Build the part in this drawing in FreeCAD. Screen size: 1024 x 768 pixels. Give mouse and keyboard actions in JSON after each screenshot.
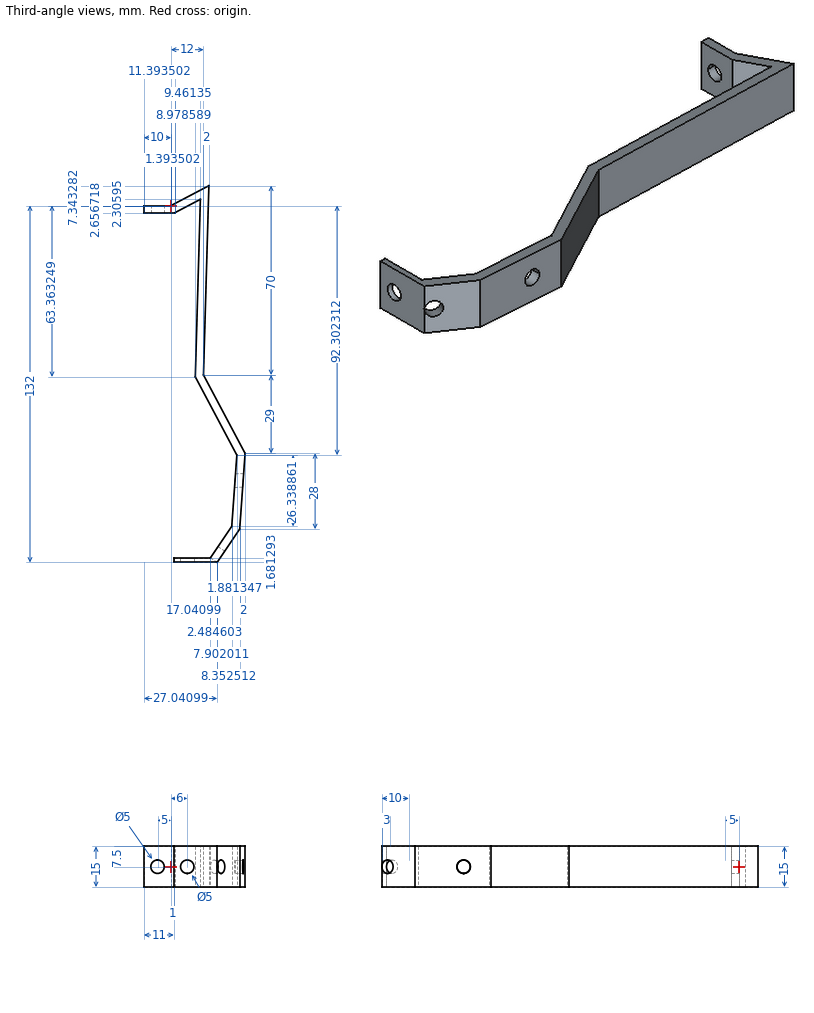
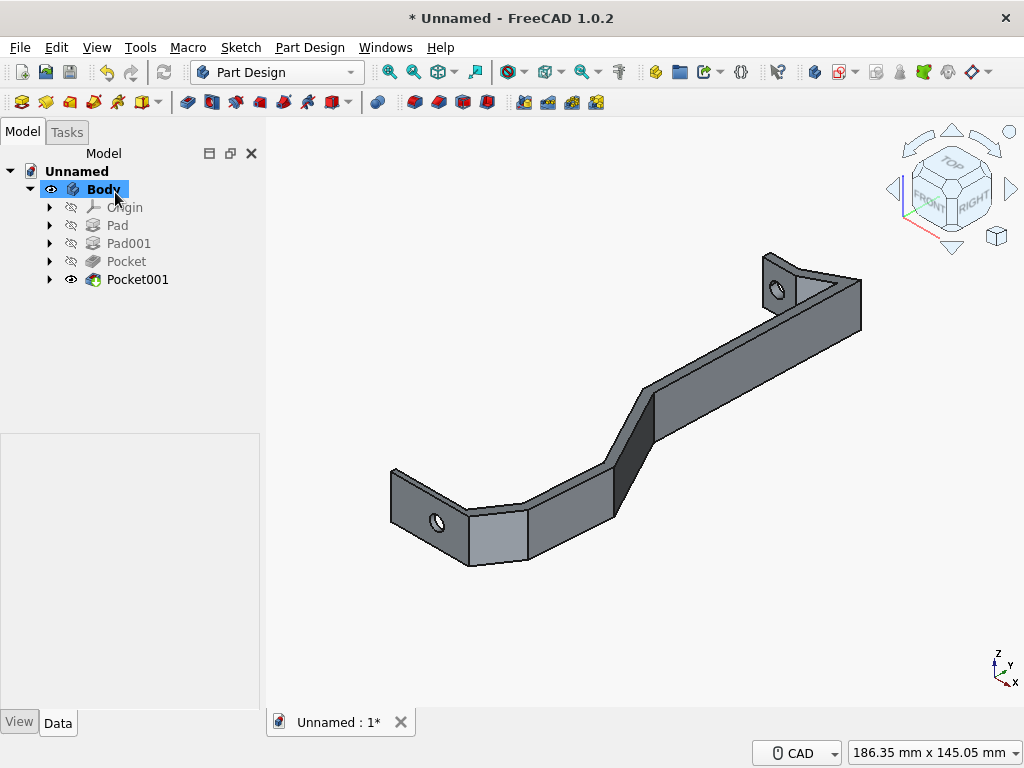
{"action": "left_click", "coordinate": [408, 505]}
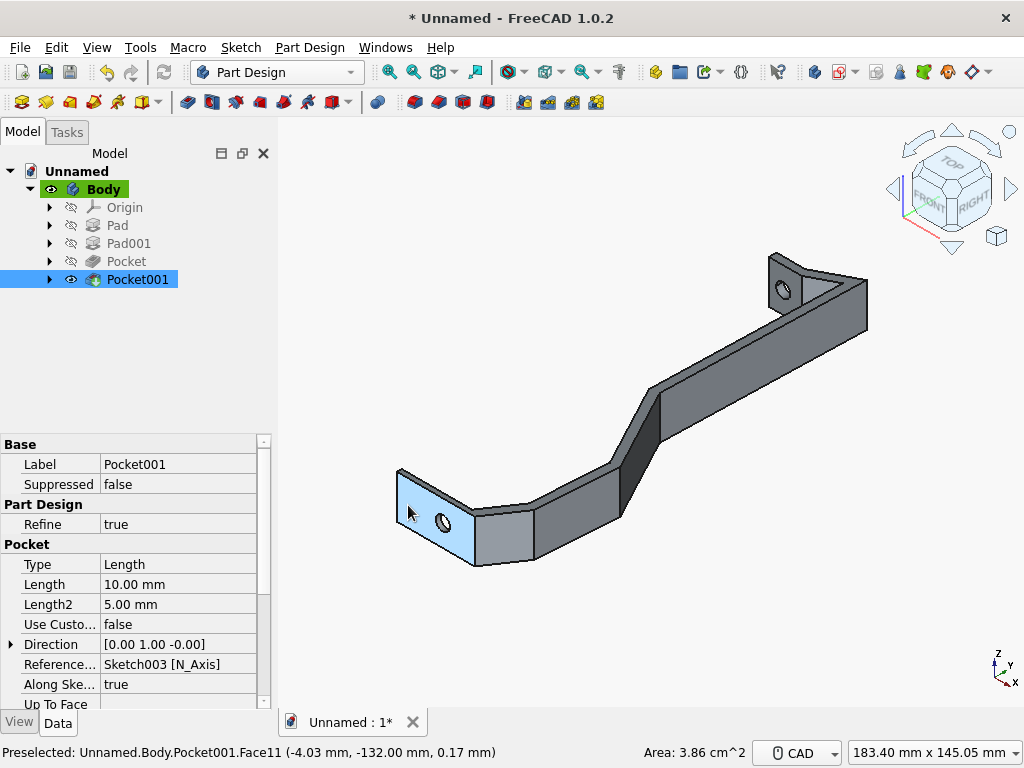
{"action": "left_click", "coordinate": [840, 72]}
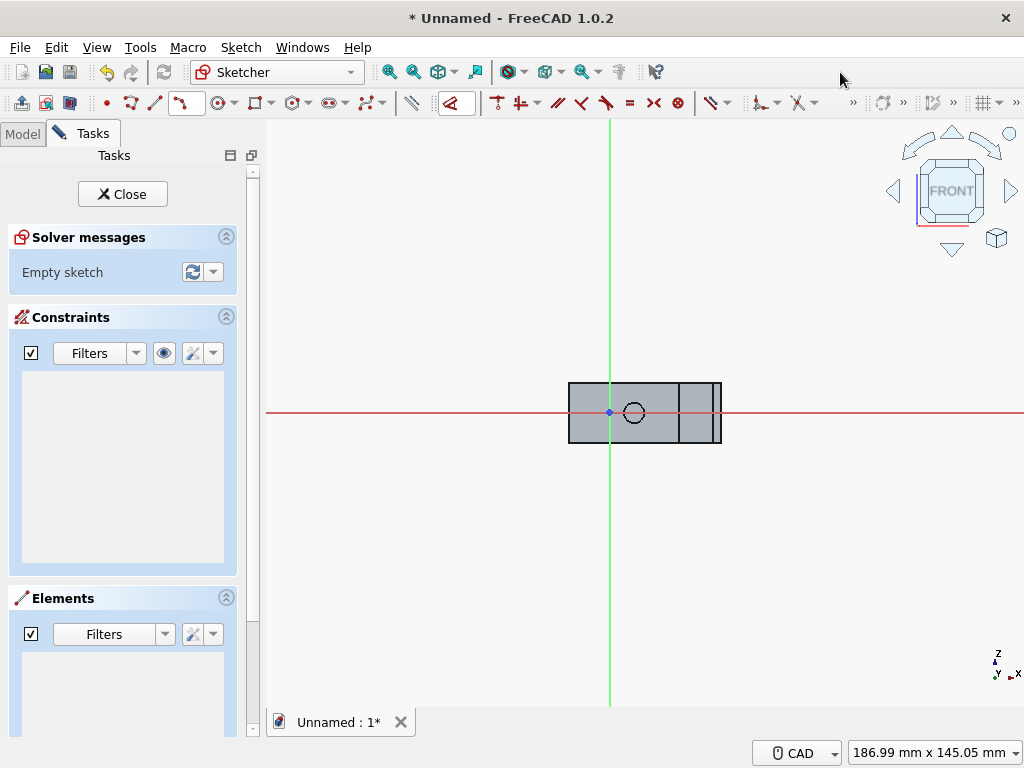
{"action": "scroll", "coordinate": [594, 413], "scroll_direction": "up", "scroll_amount": 9}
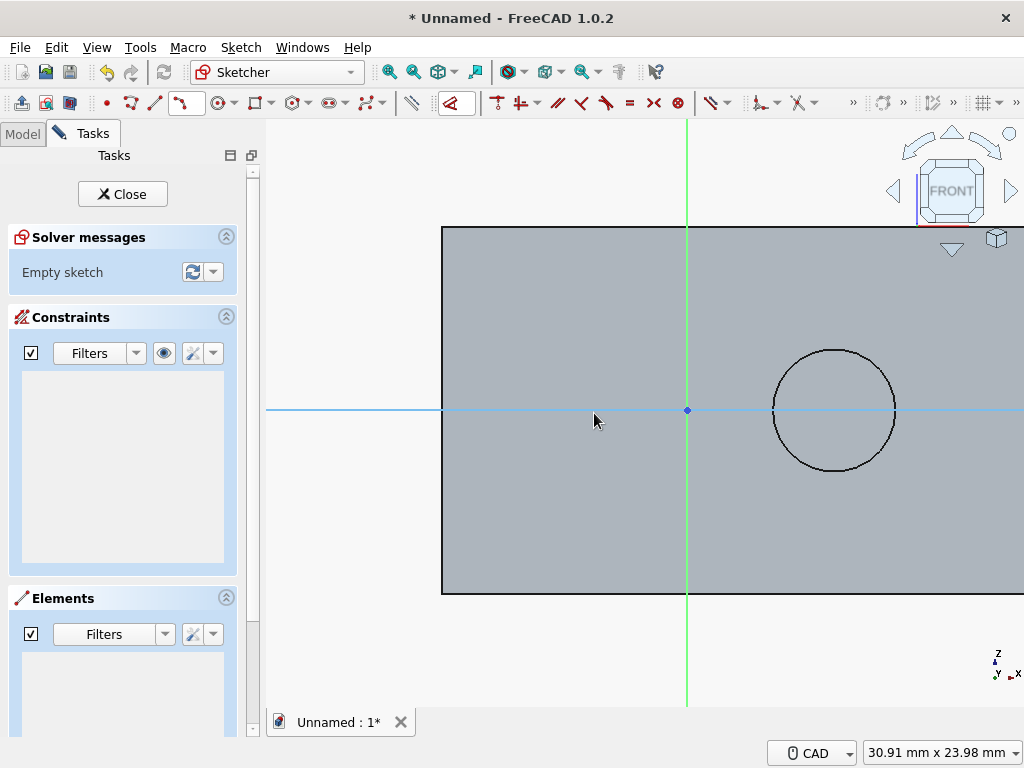
{"action": "left_click", "coordinate": [256, 104]}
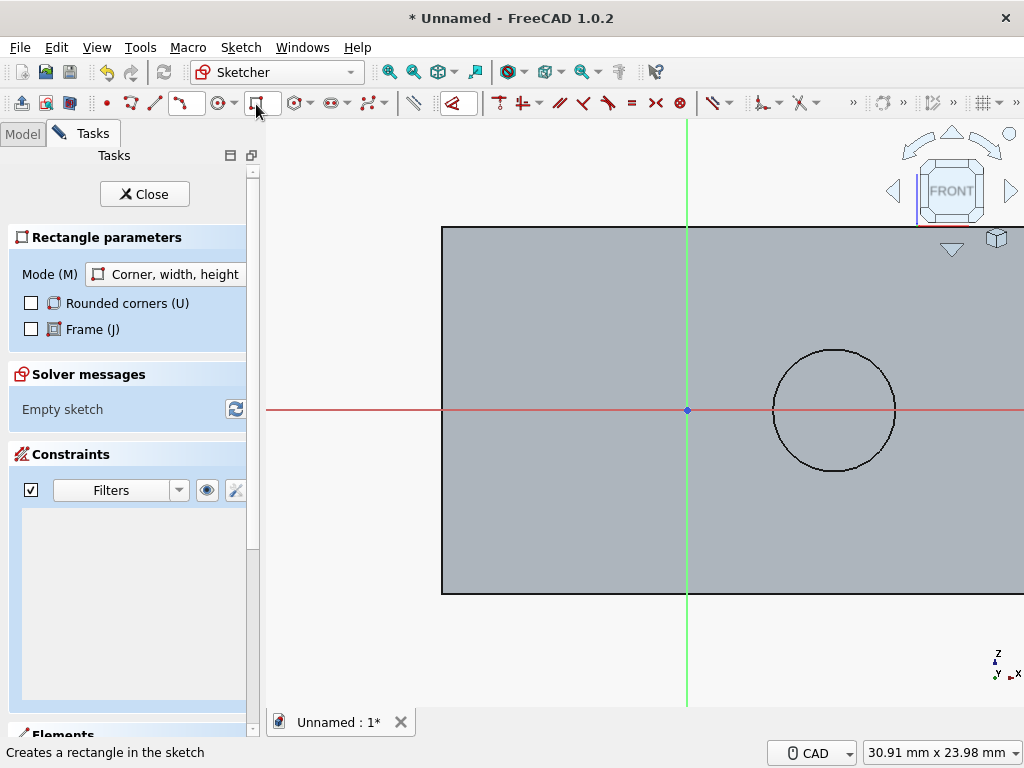
{"action": "left_click", "coordinate": [442, 227]}
{"action": "mouse_move", "coordinate": [712, 594]}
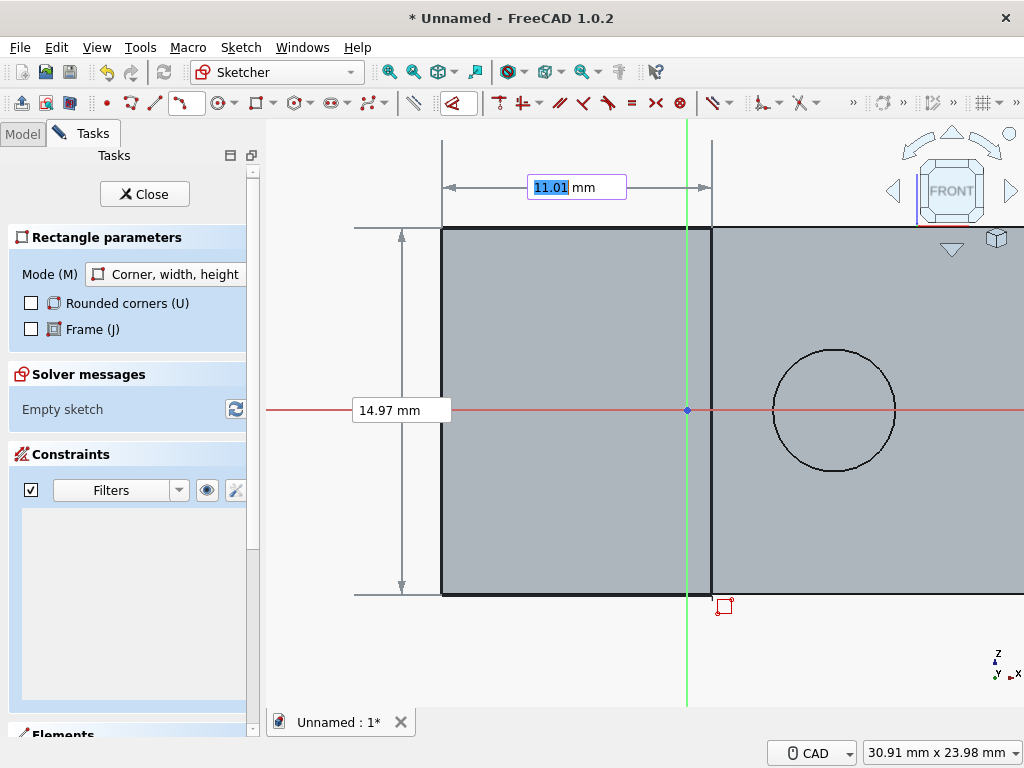
{"action": "type", "text": "11"}
{"action": "key", "text": "Tab"}
{"action": "type", "text": "15"}
{"action": "key", "text": "Return"}
{"action": "key", "text": "Escape"}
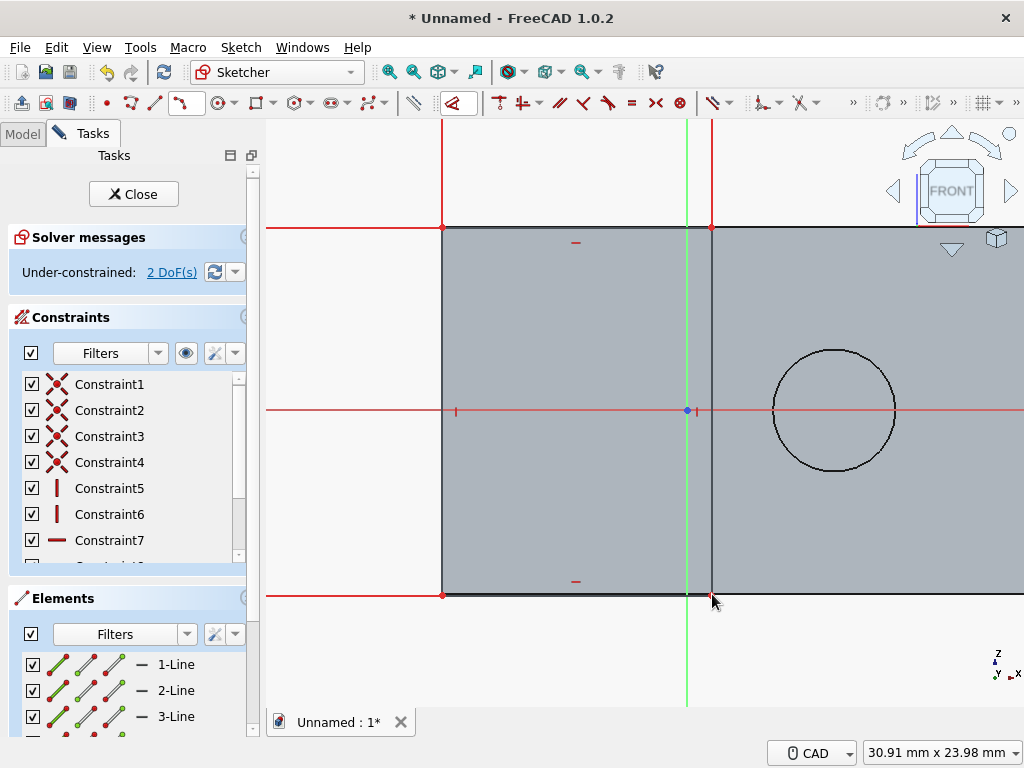
{"action": "scroll", "coordinate": [712, 596], "scroll_direction": "up", "scroll_amount": 3}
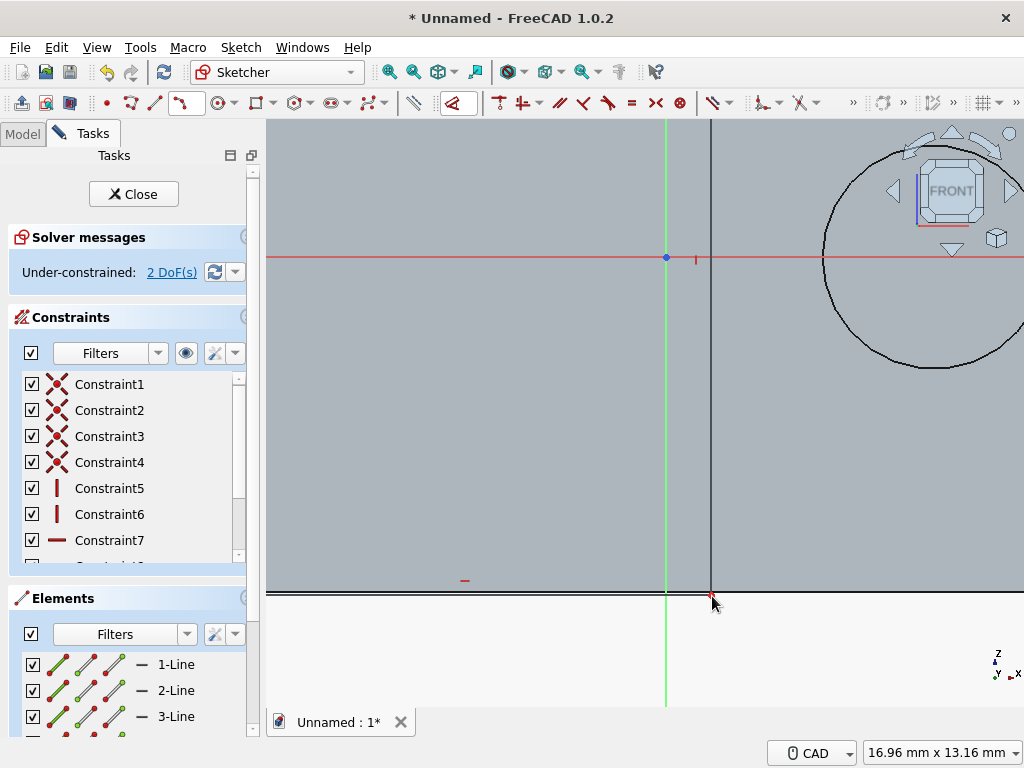
{"action": "left_click", "coordinate": [711, 595]}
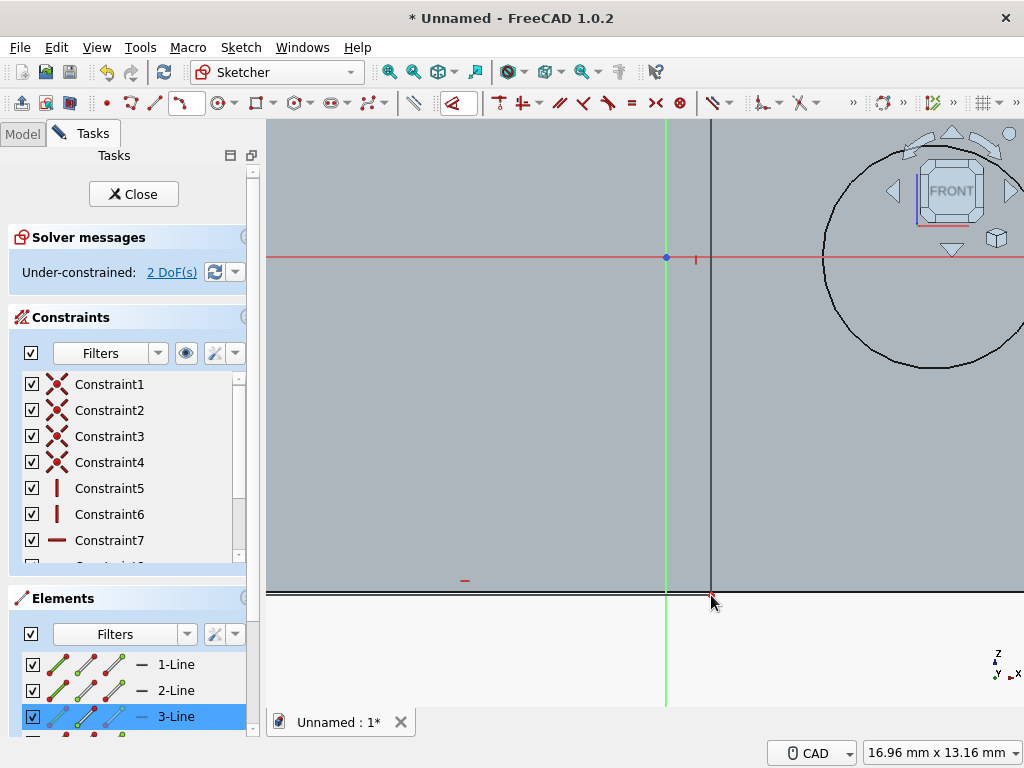
{"action": "left_click", "coordinate": [472, 104]}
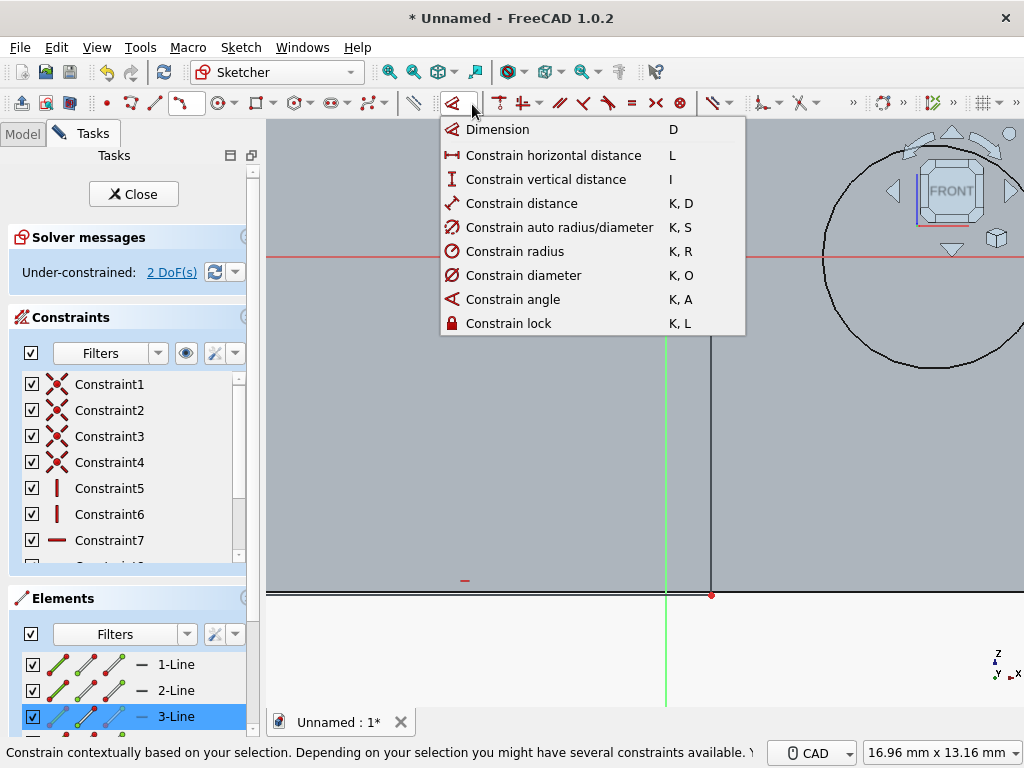
{"action": "left_click", "coordinate": [593, 155]}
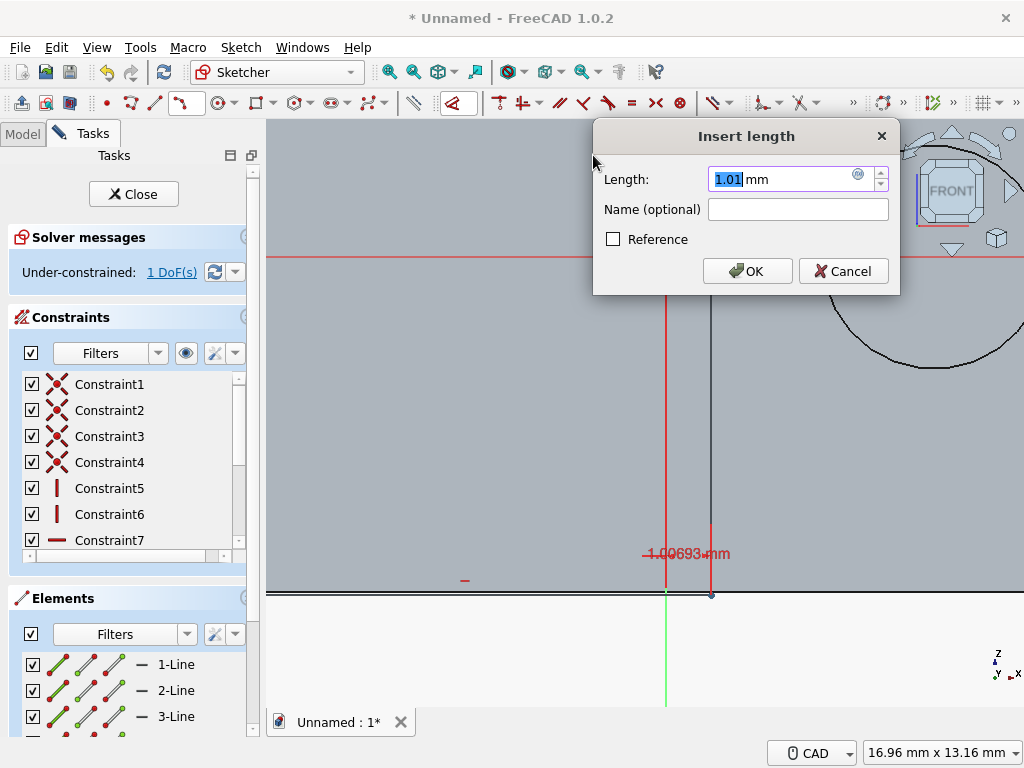
{"action": "type", "text": "1"}
{"action": "key", "text": "Return"}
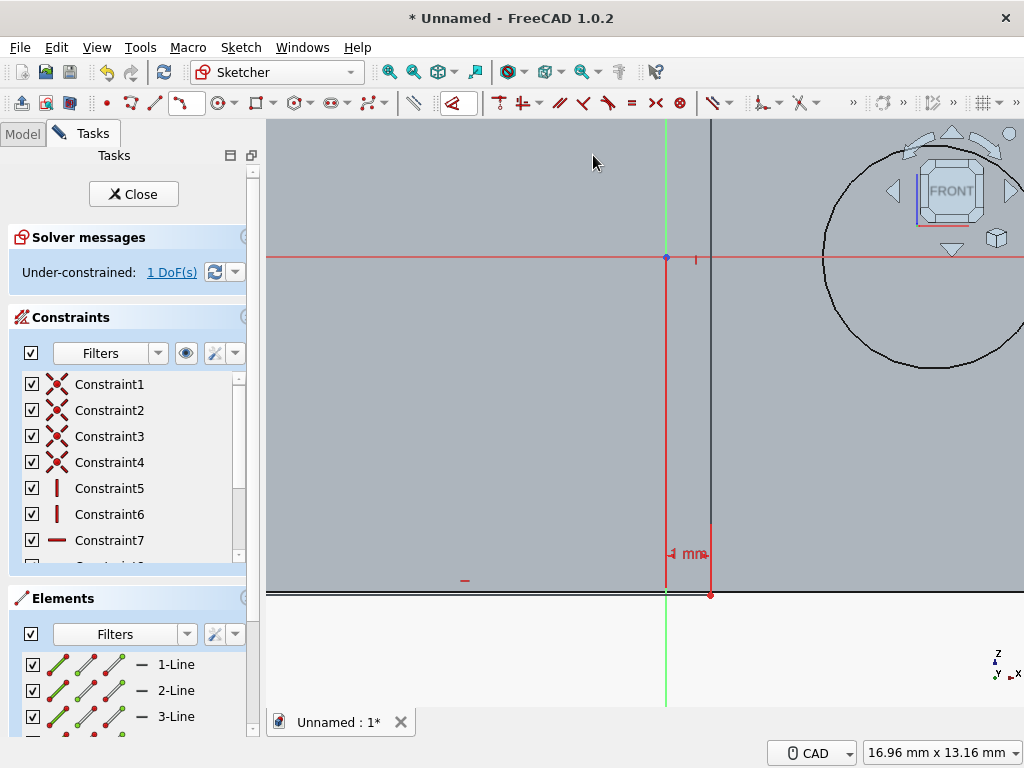
{"action": "scroll", "coordinate": [712, 602], "scroll_direction": "down", "scroll_amount": 3}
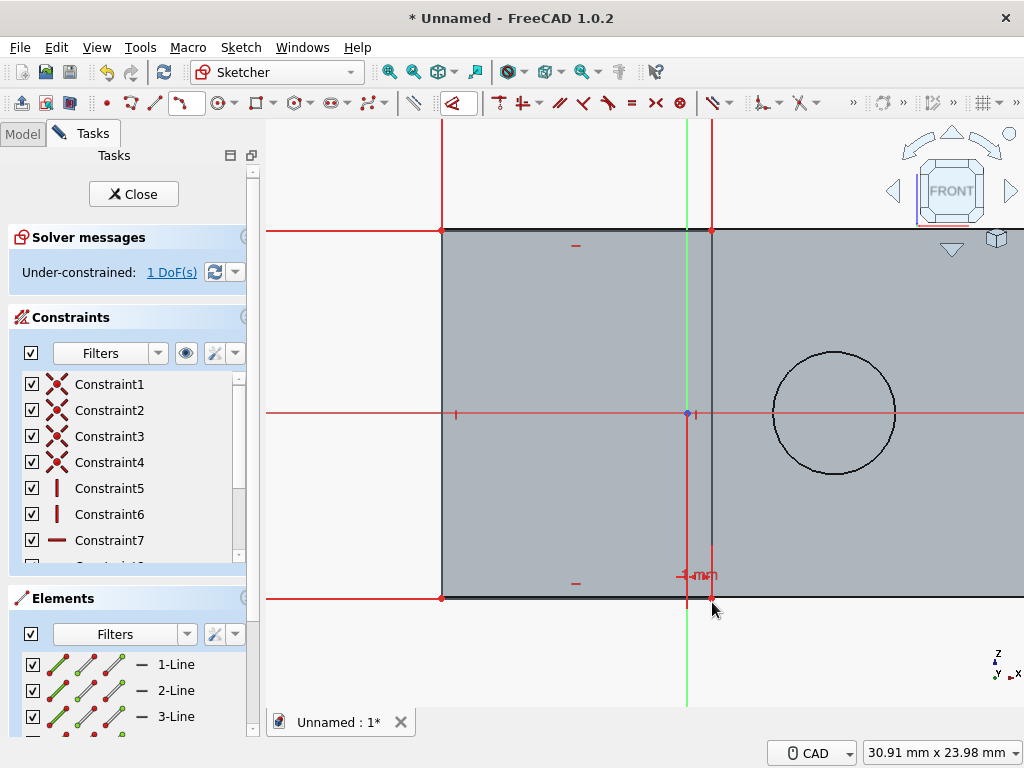
{"action": "left_click", "coordinate": [442, 231]}